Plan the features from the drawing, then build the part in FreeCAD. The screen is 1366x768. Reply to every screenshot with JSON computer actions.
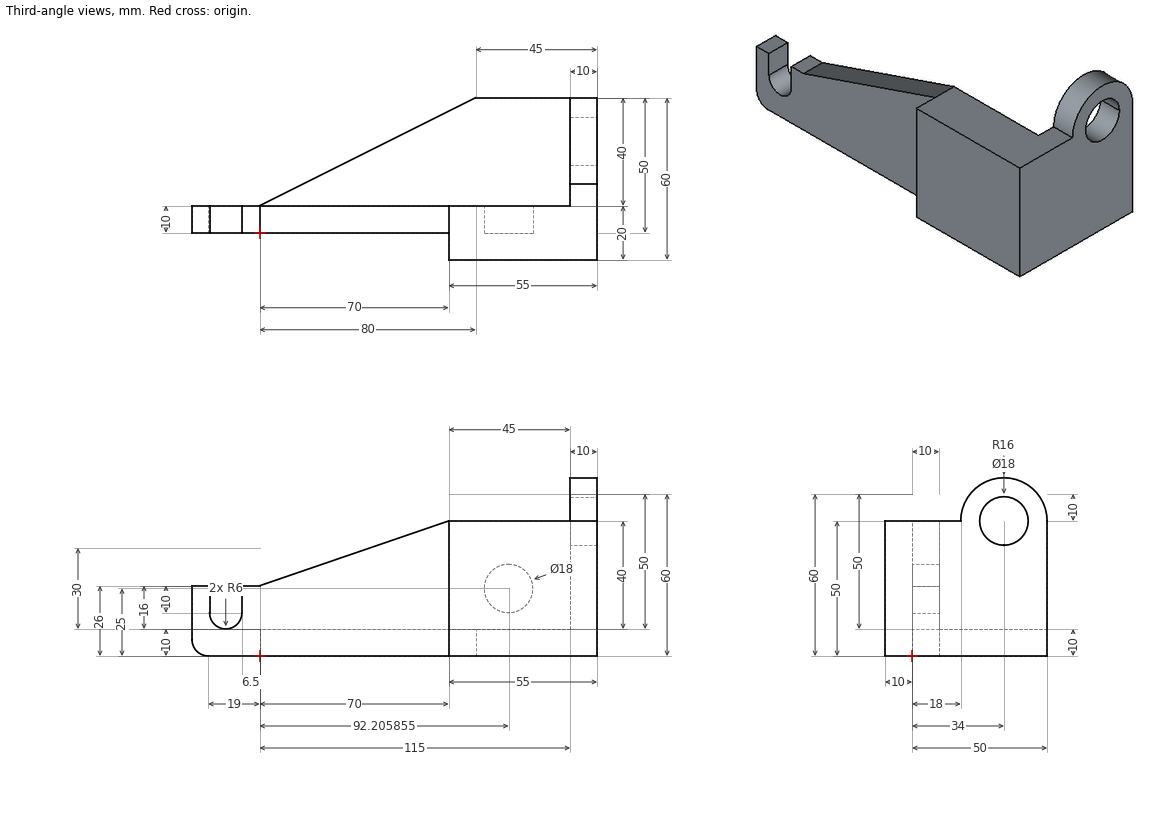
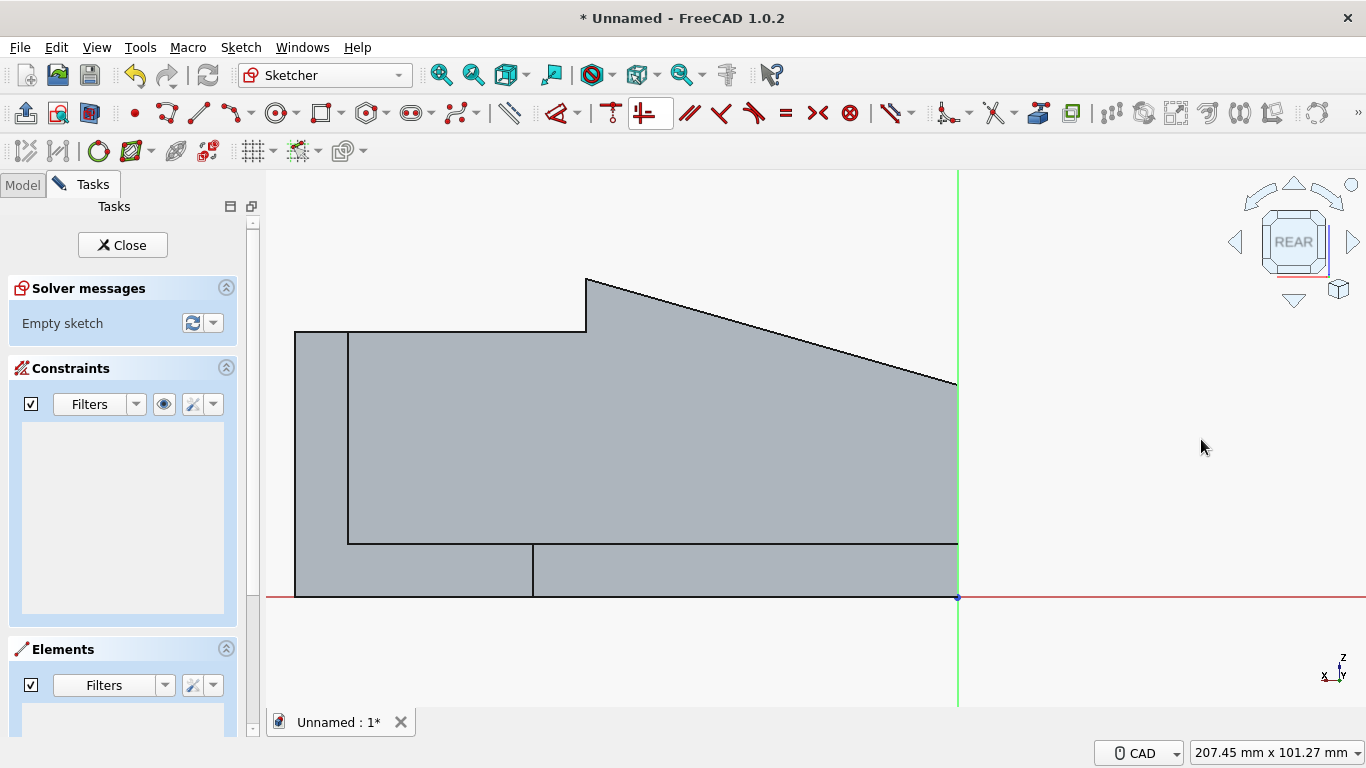
{"action": "left_click", "coordinate": [168, 114]}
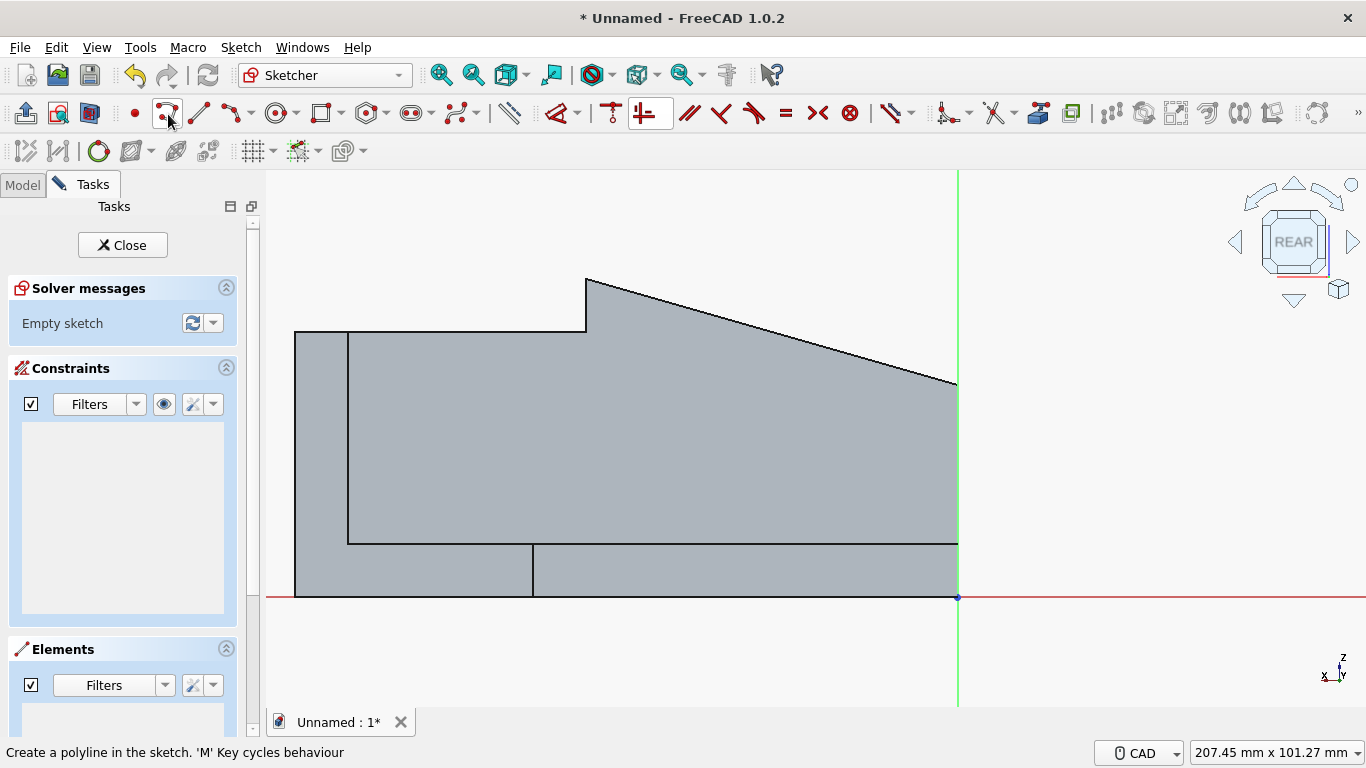
{"action": "left_click", "coordinate": [958, 544]}
{"action": "left_click", "coordinate": [949, 385]}
{"action": "left_click", "coordinate": [586, 279]}
{"action": "left_click", "coordinate": [586, 544]}
{"action": "left_click", "coordinate": [958, 545]}
{"action": "key", "text": "Escape"}
{"action": "key", "text": "Escape"}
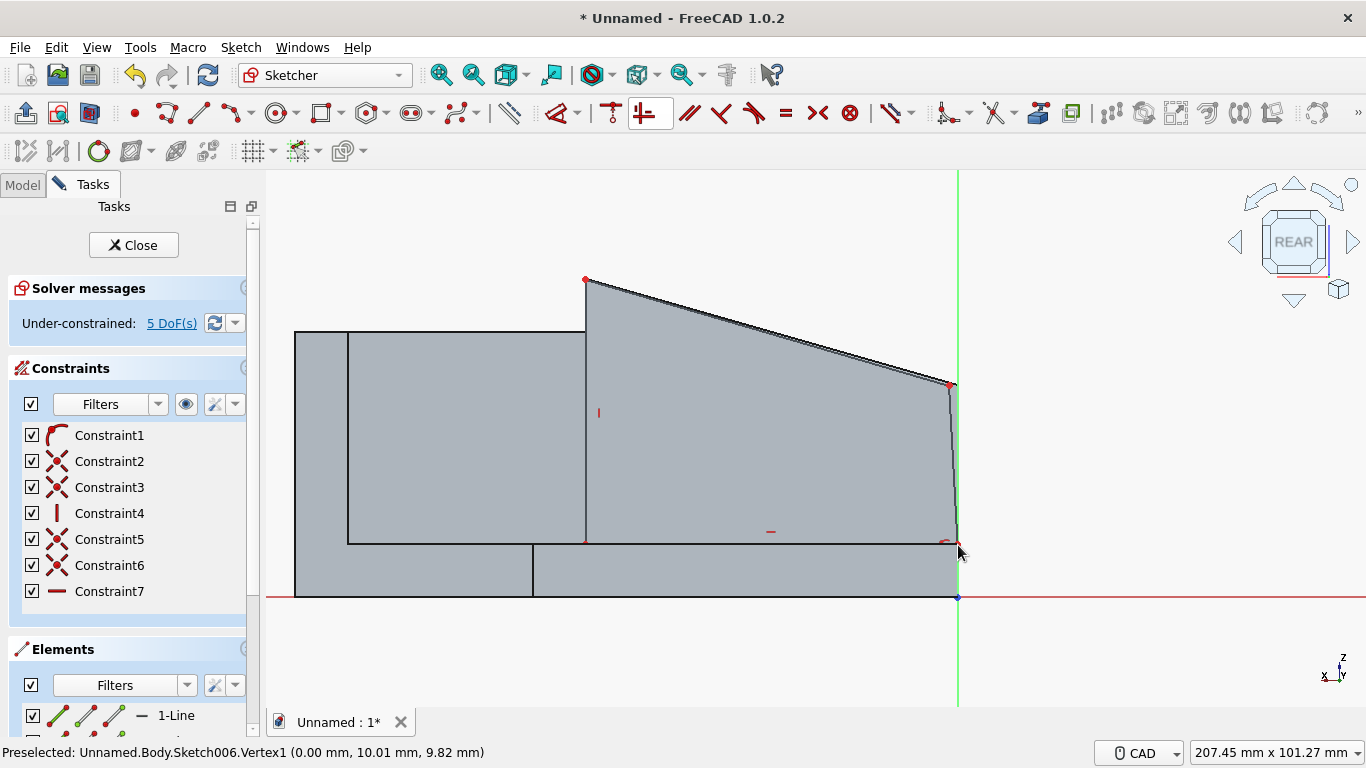
{"action": "left_click", "coordinate": [955, 497]}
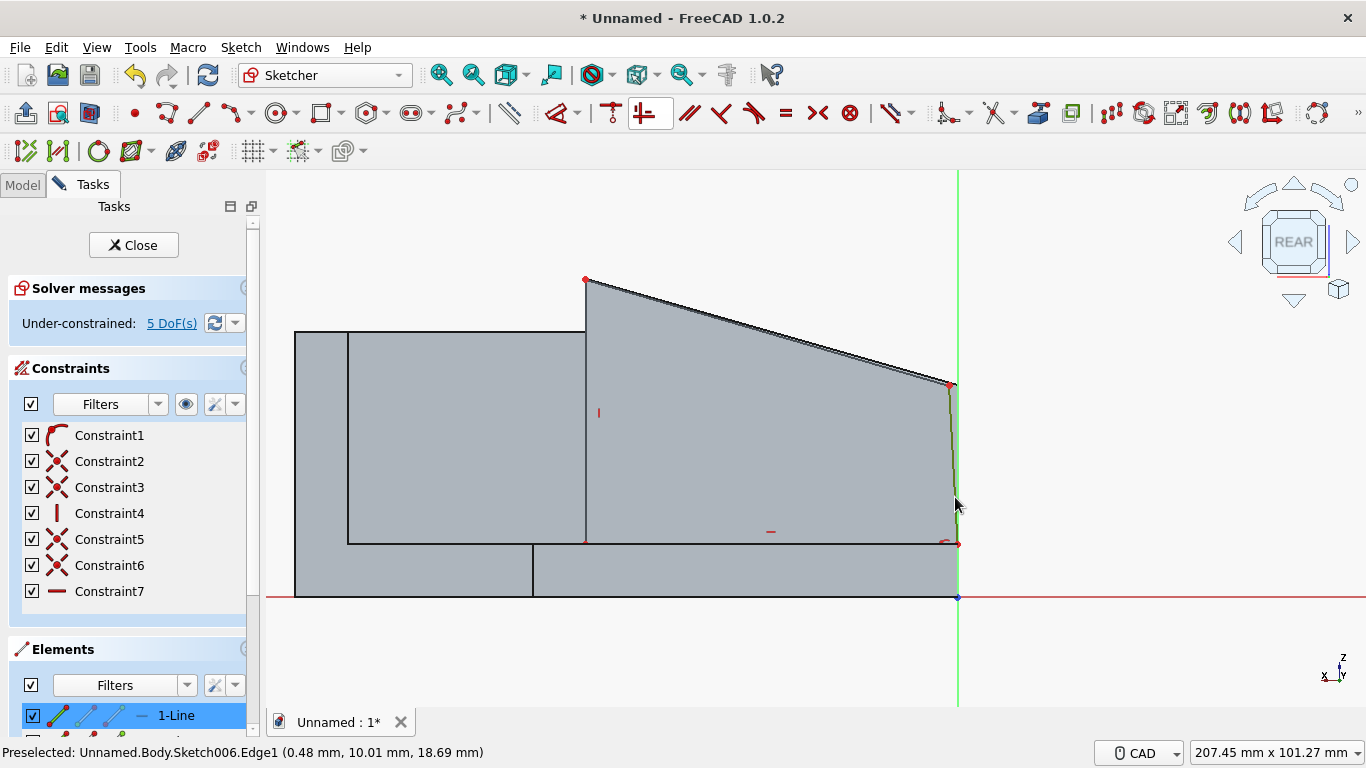
{"action": "key", "text": "v"}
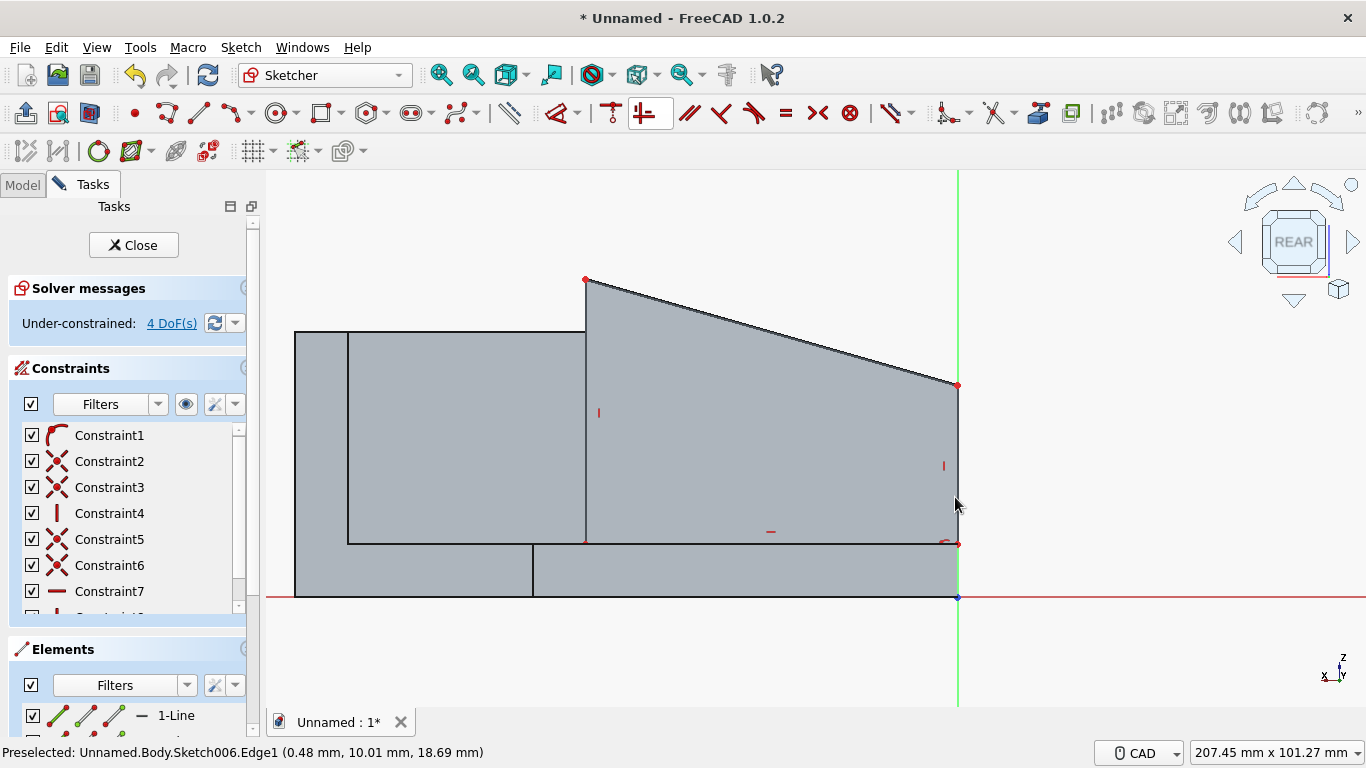
{"action": "left_click", "coordinate": [556, 114]}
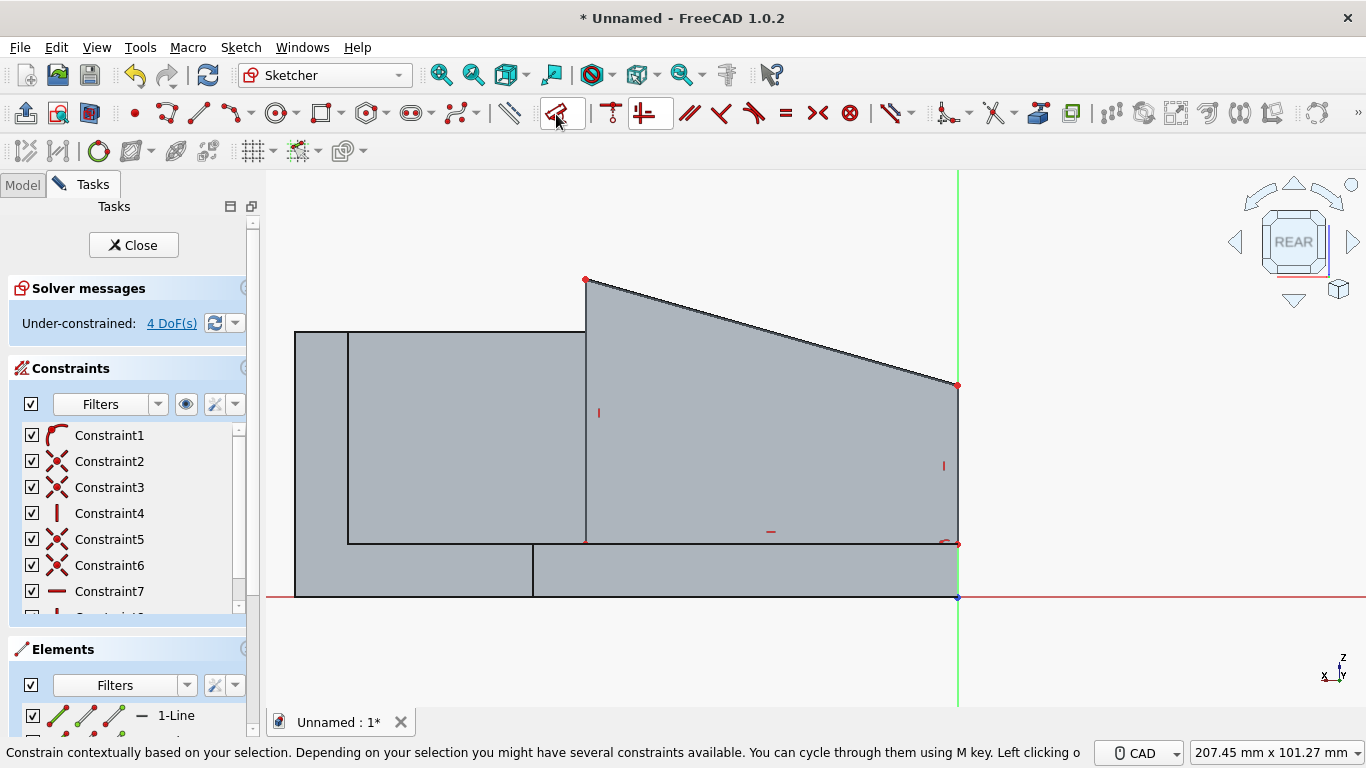
{"action": "left_click", "coordinate": [958, 497]}
{"action": "left_click", "coordinate": [992, 465]}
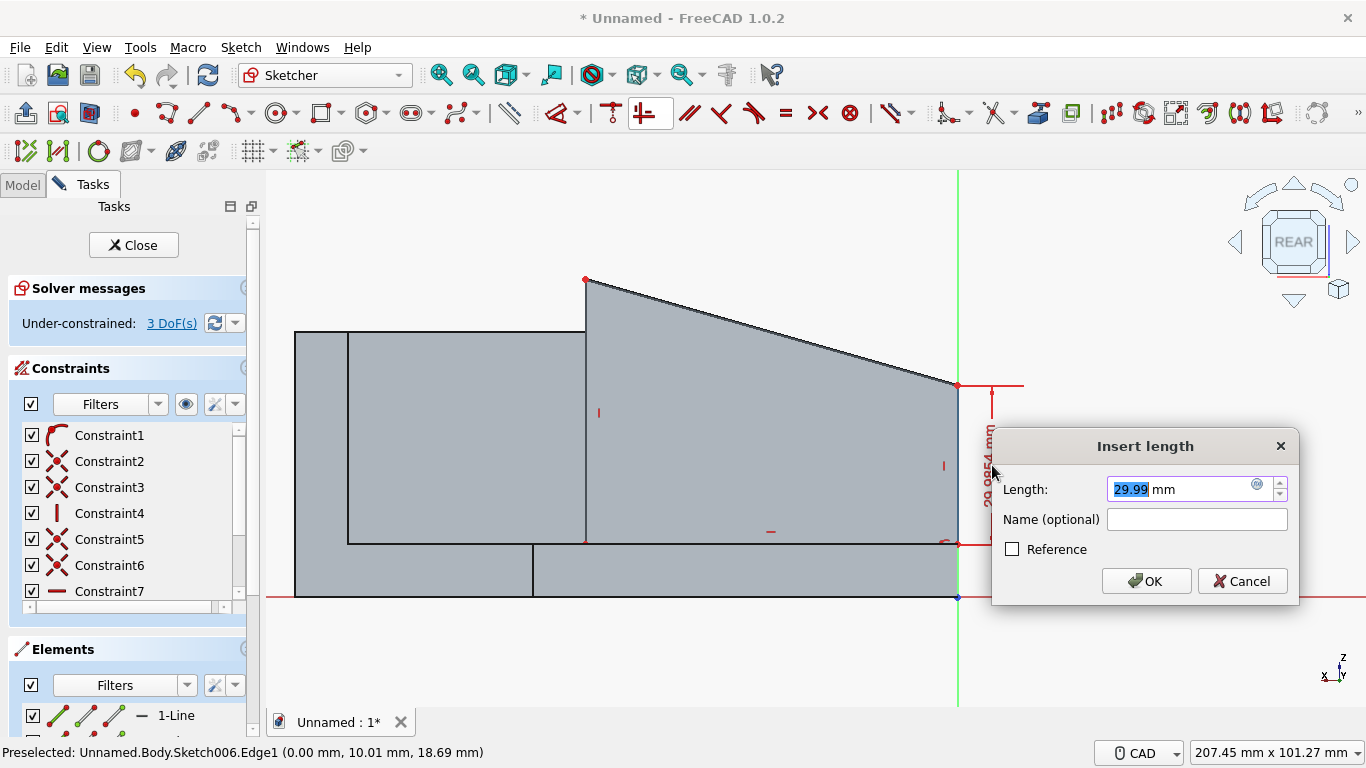
{"action": "type", "text": "30"}
{"action": "key", "text": "Return"}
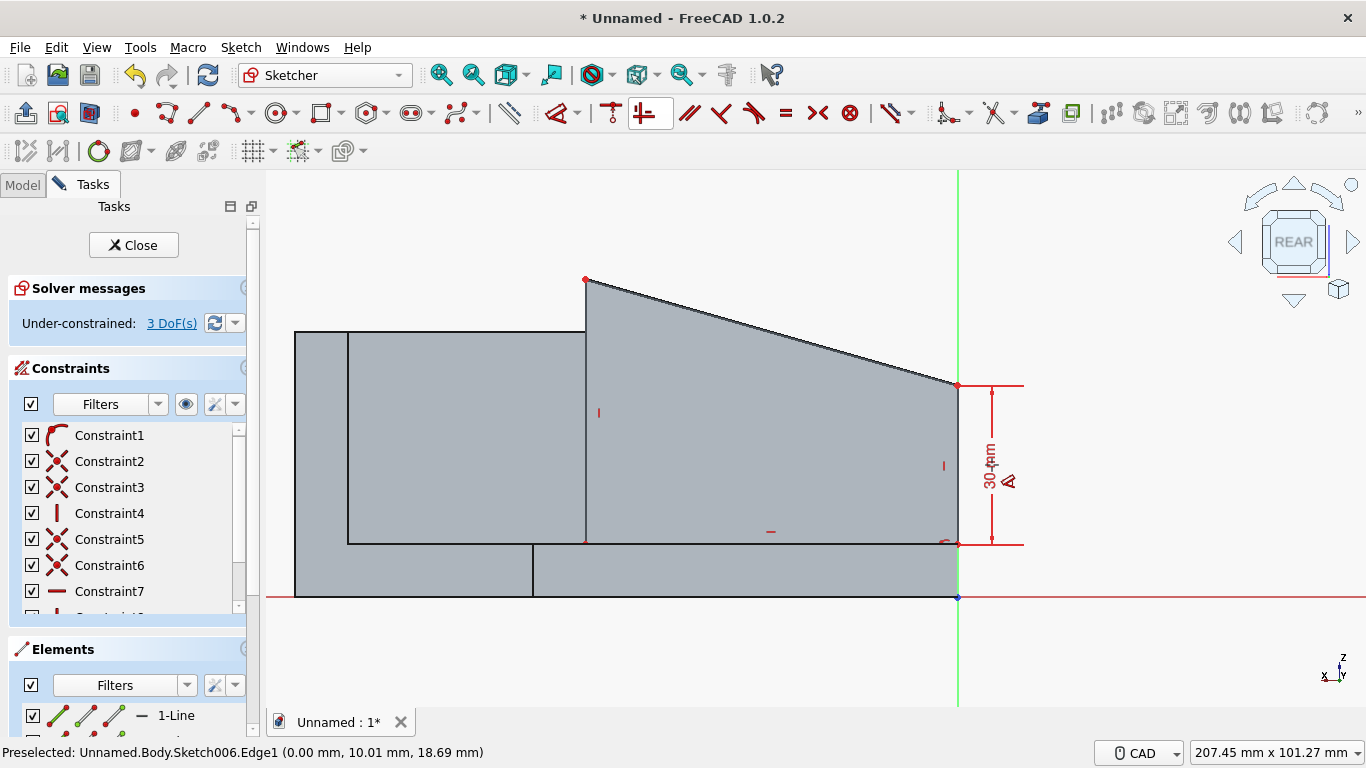
{"action": "left_click", "coordinate": [586, 360]}
{"action": "left_click", "coordinate": [552, 413]}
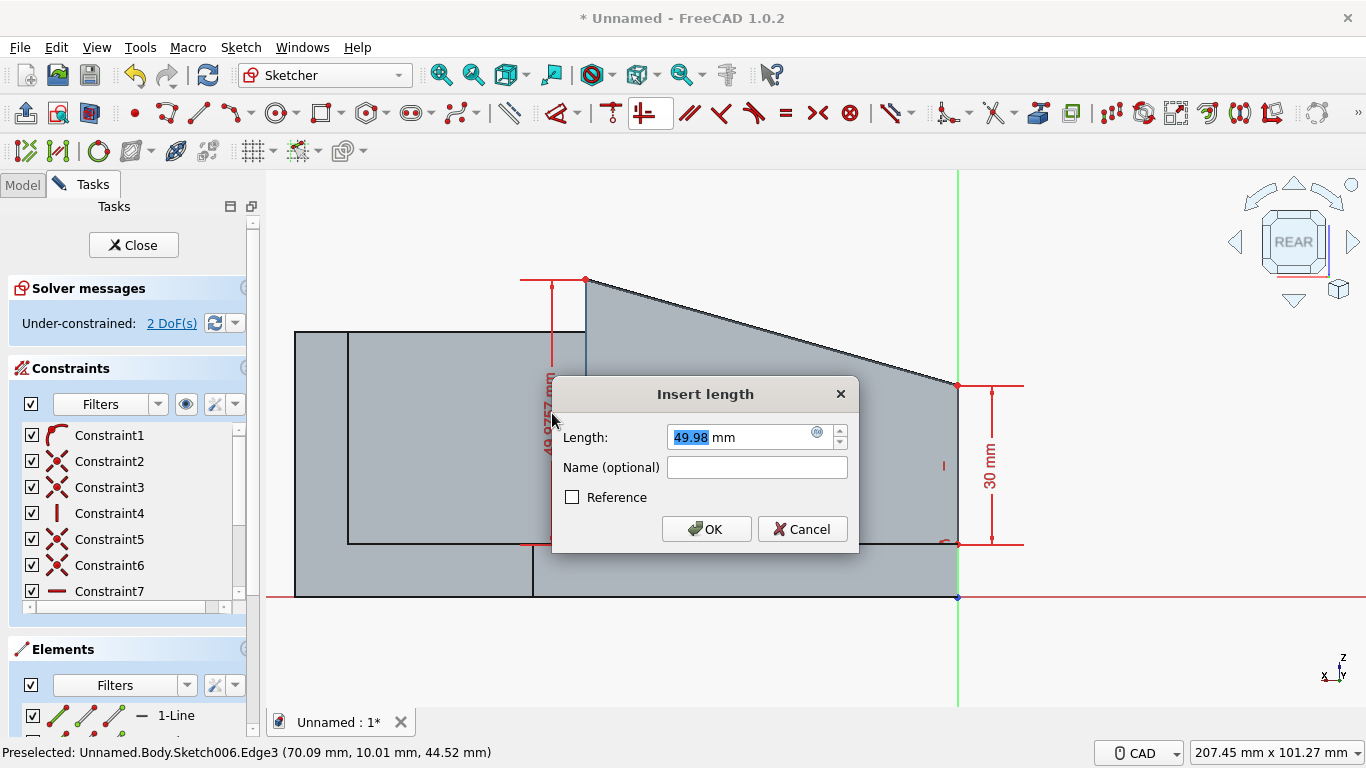
{"action": "type", "text": "50"}
{"action": "key", "text": "Return"}